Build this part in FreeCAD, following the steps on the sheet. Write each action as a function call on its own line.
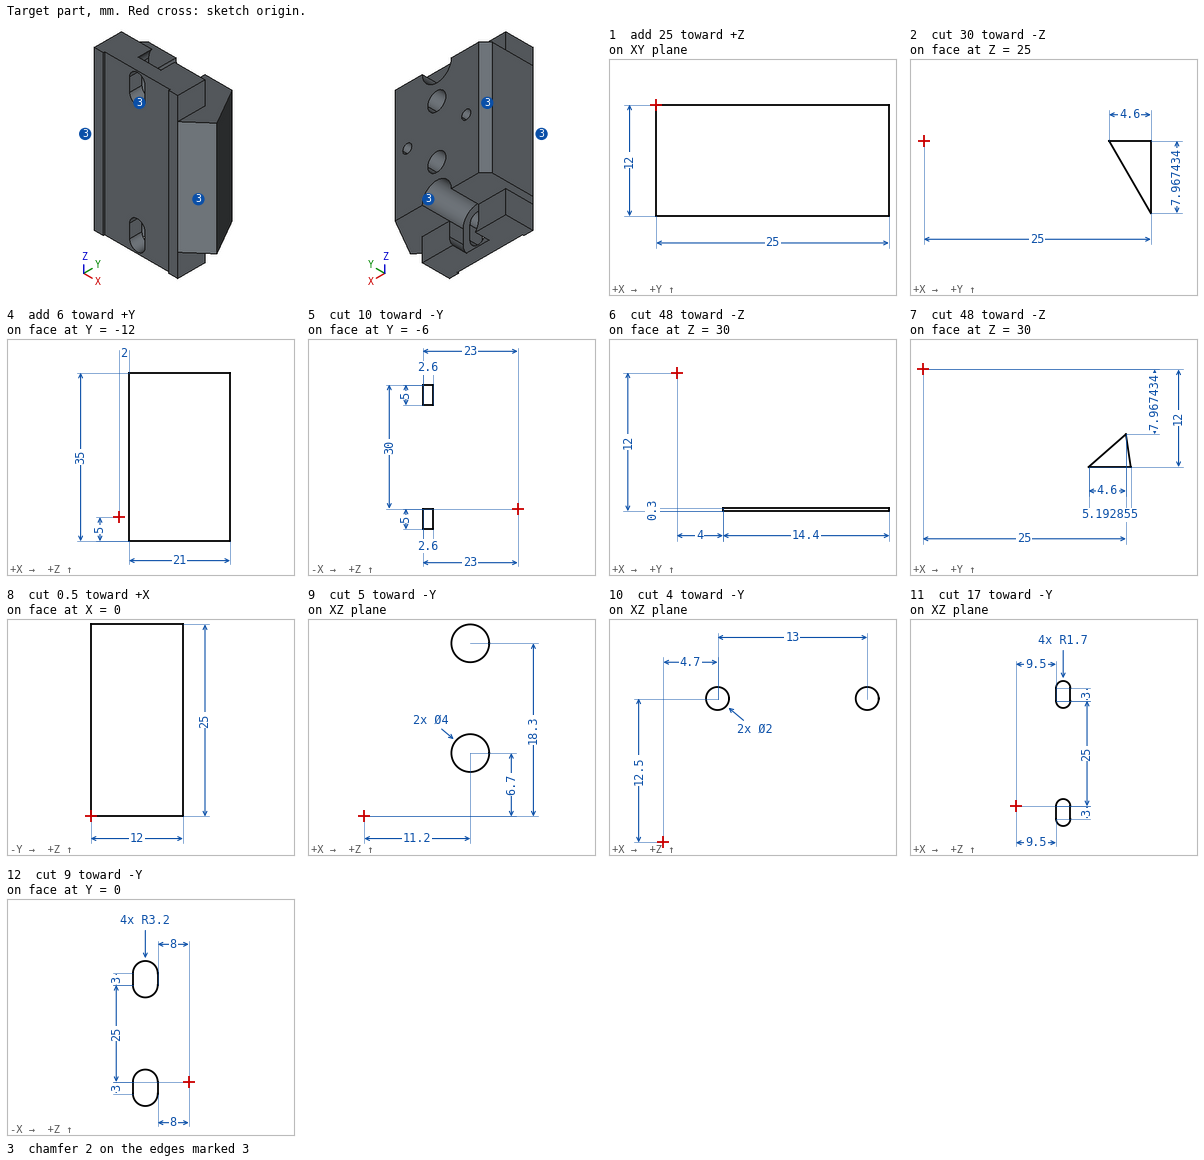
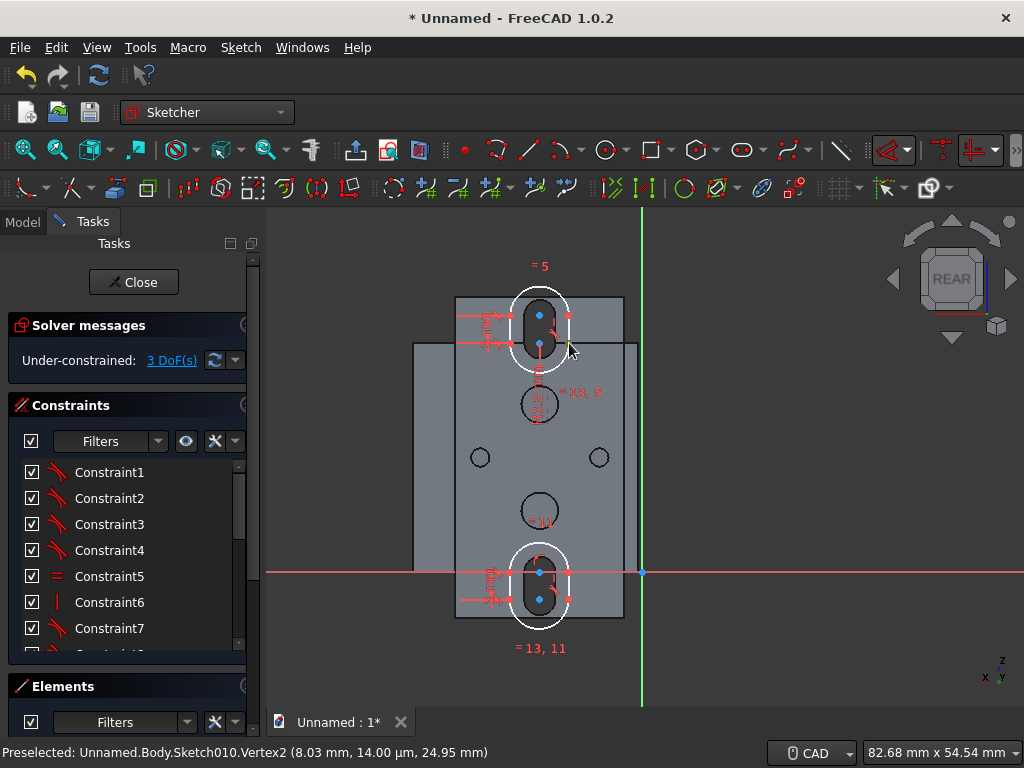
key(l)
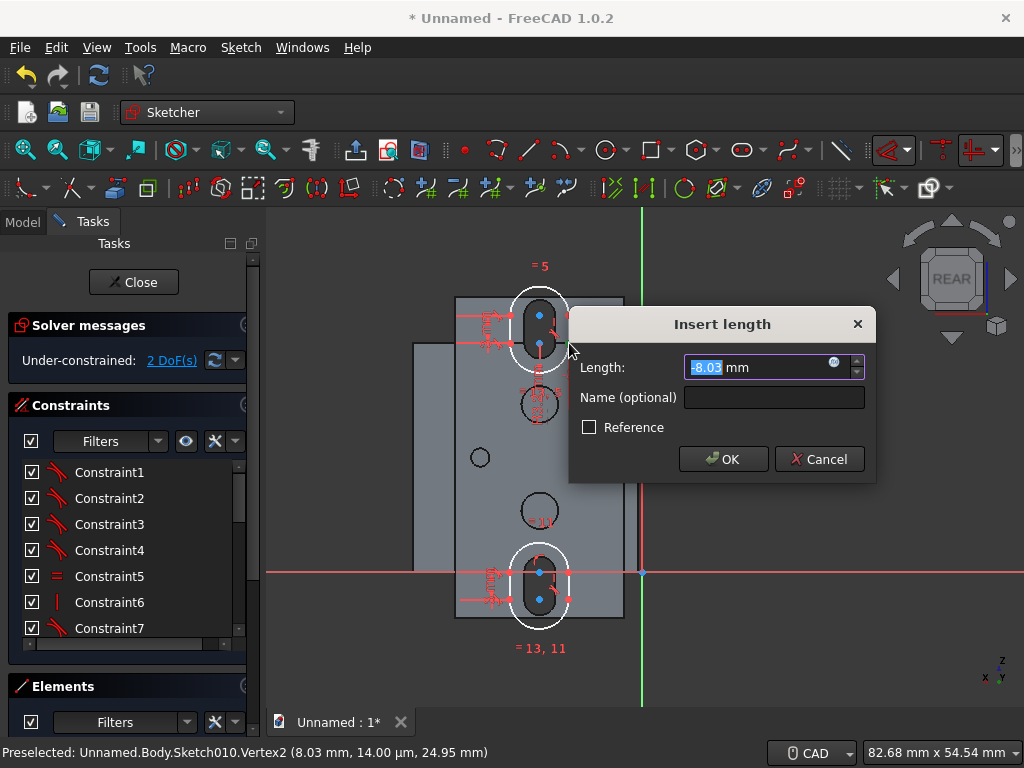
text(-8)
key(Return)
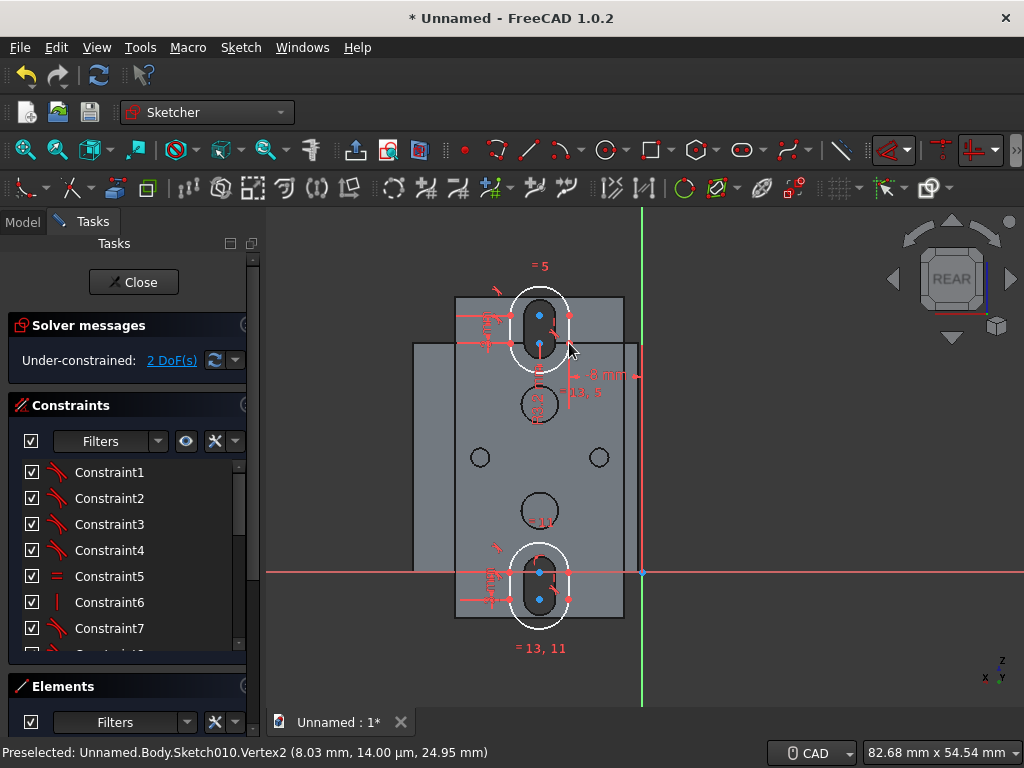
click(569, 600)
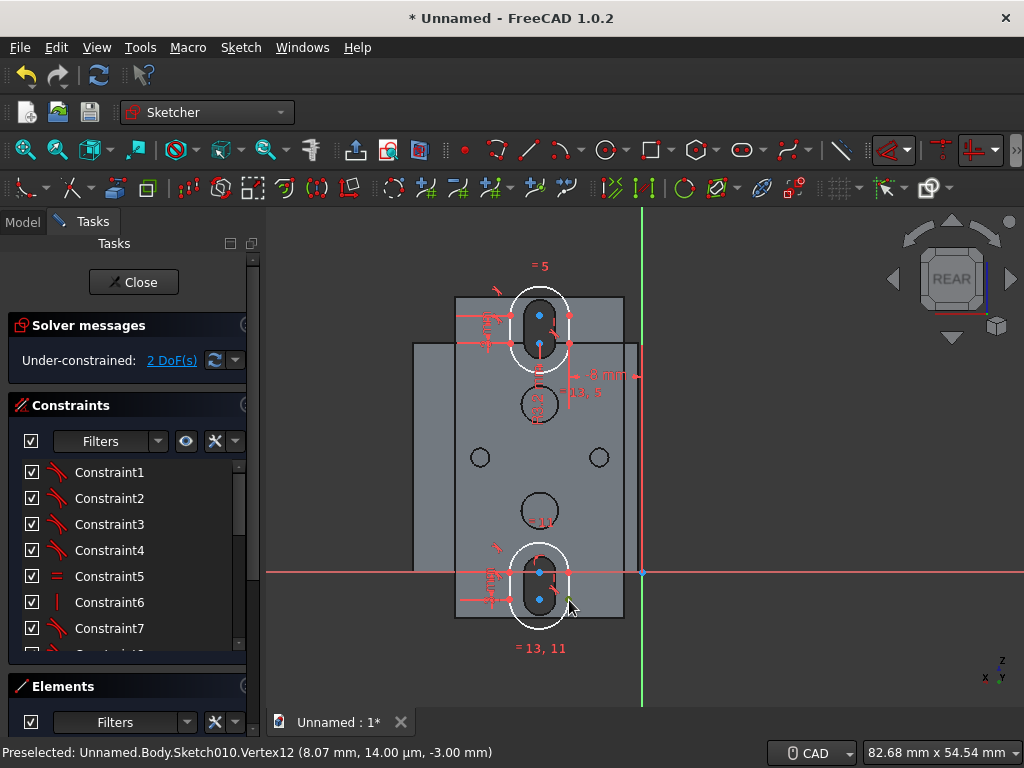
click(910, 150)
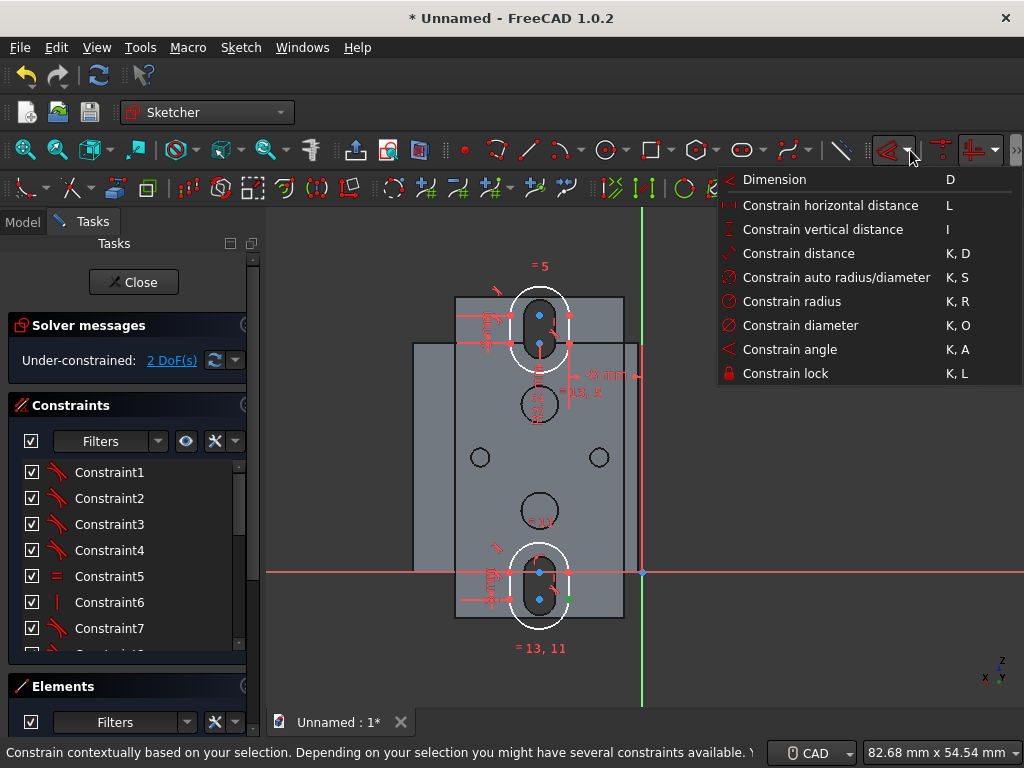
click(870, 205)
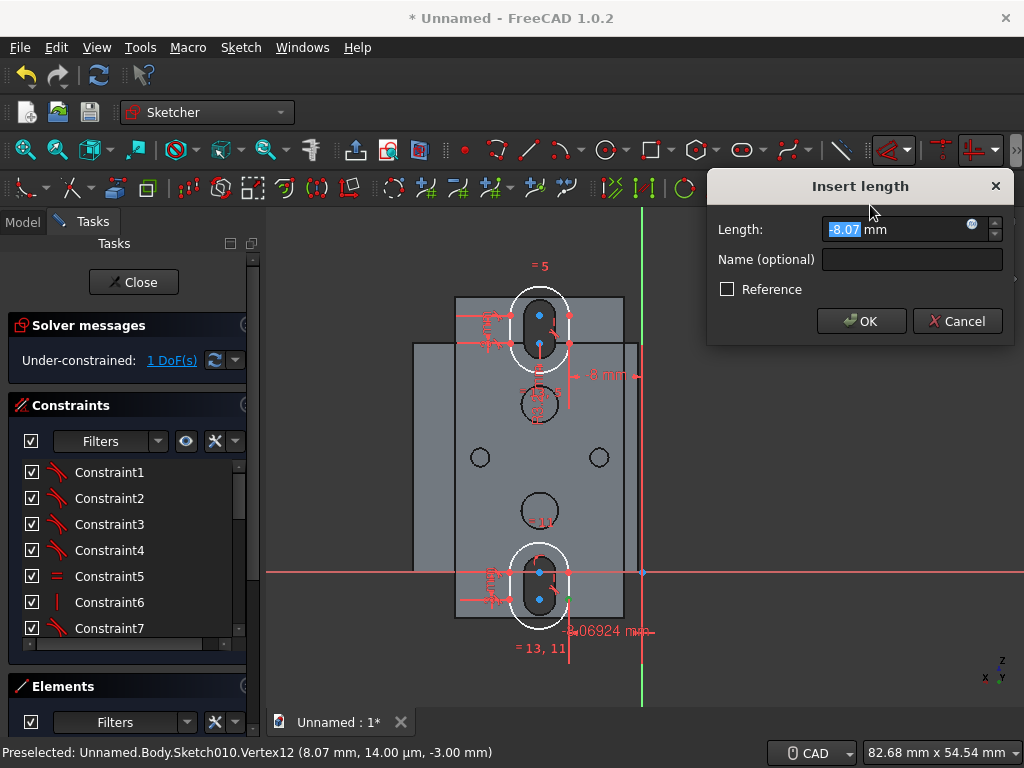
text(-8)
key(Return)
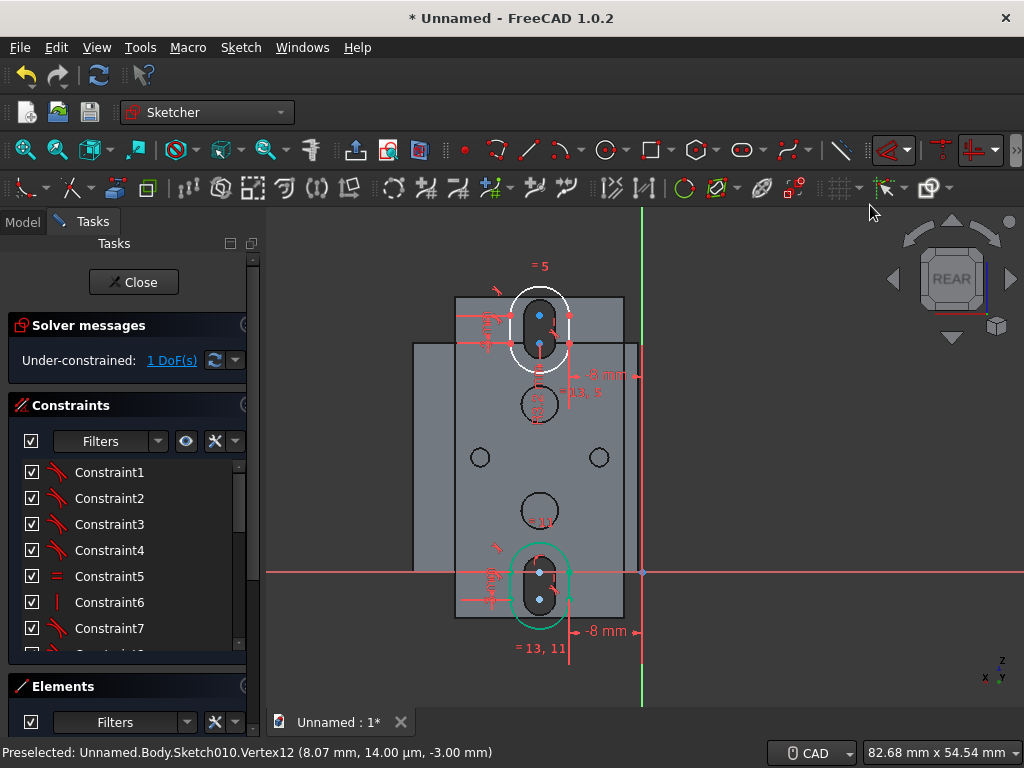
click(510, 343)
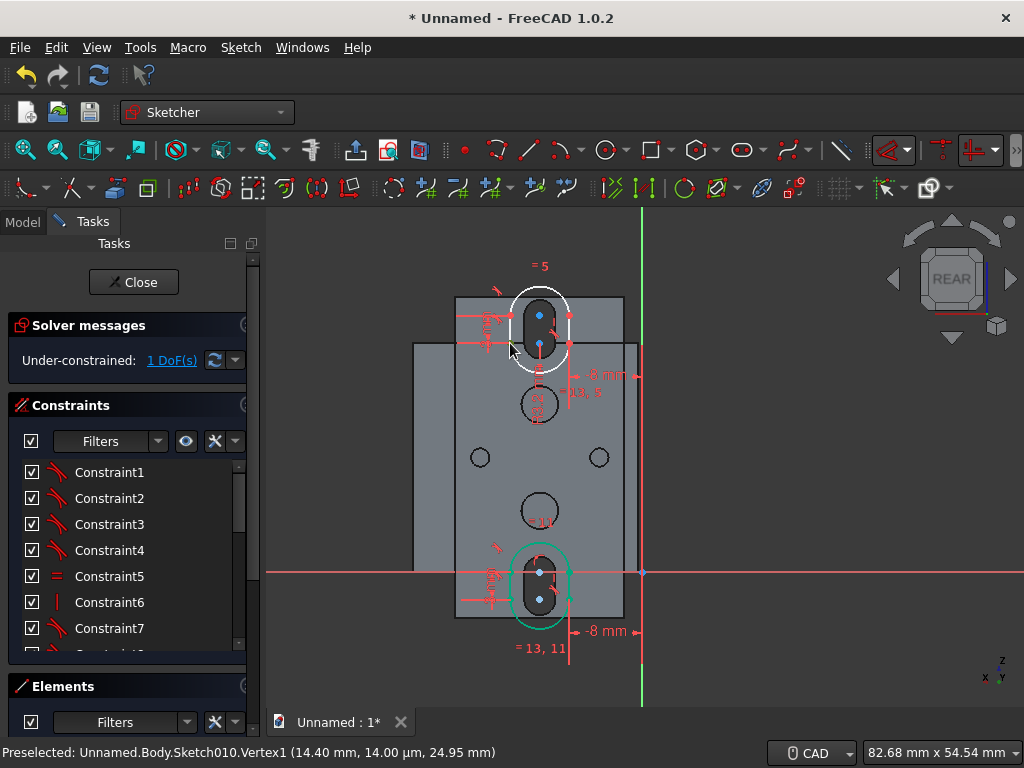
click(910, 150)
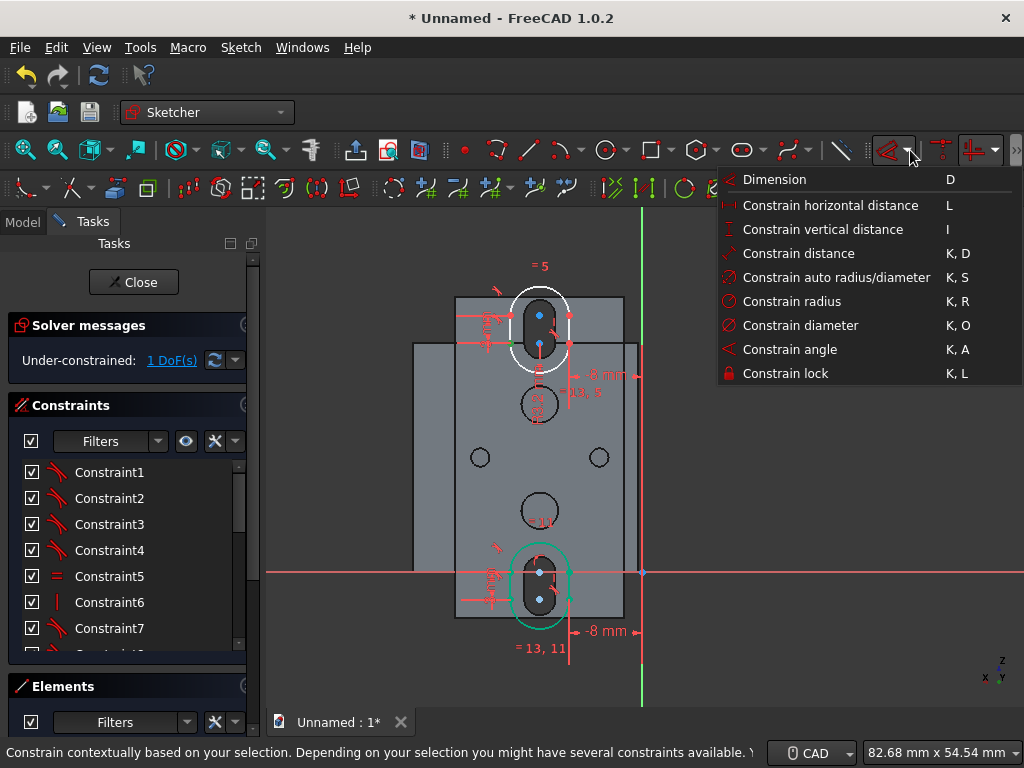
click(870, 229)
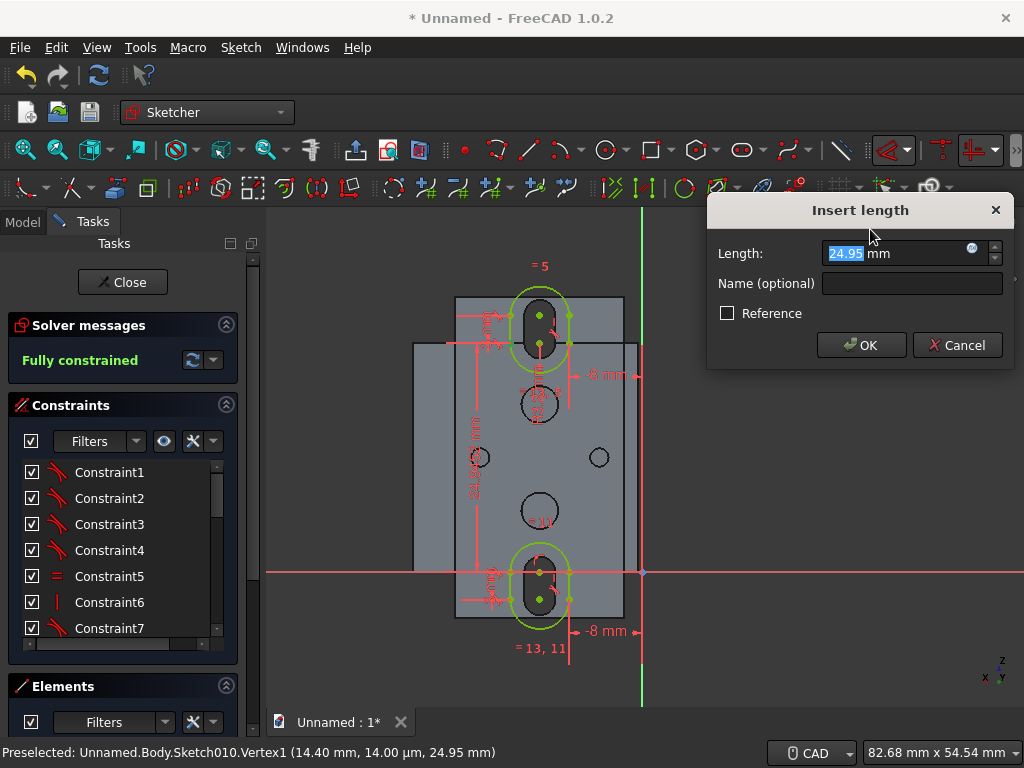
text(25)
key(Return)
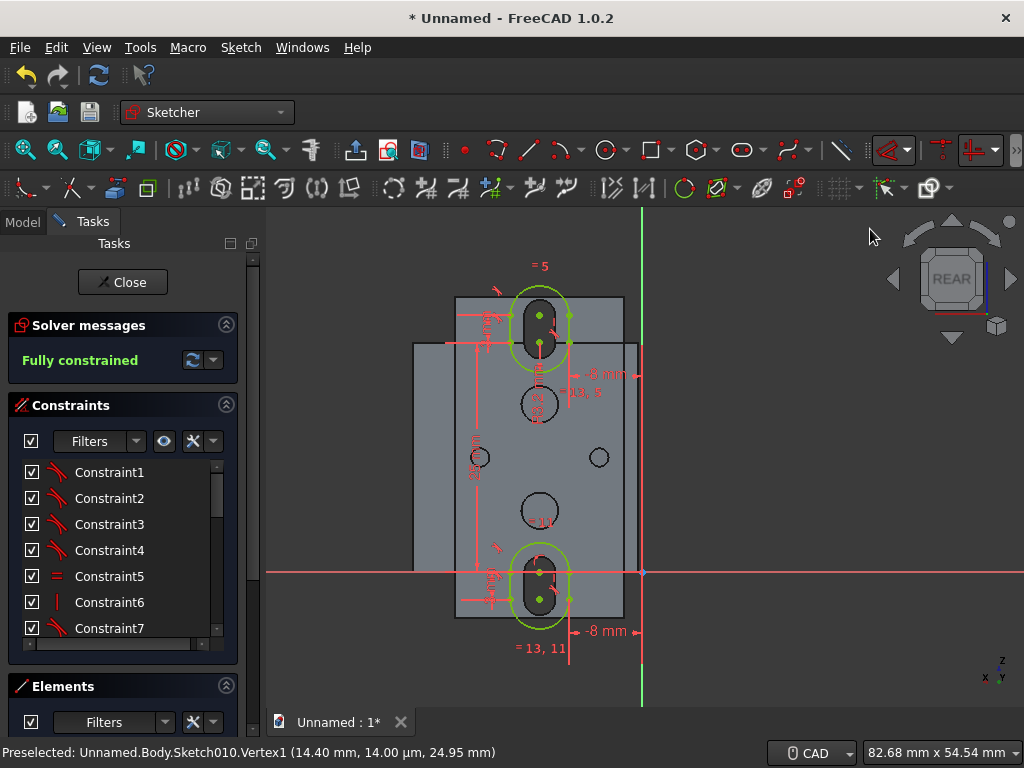
click(123, 282)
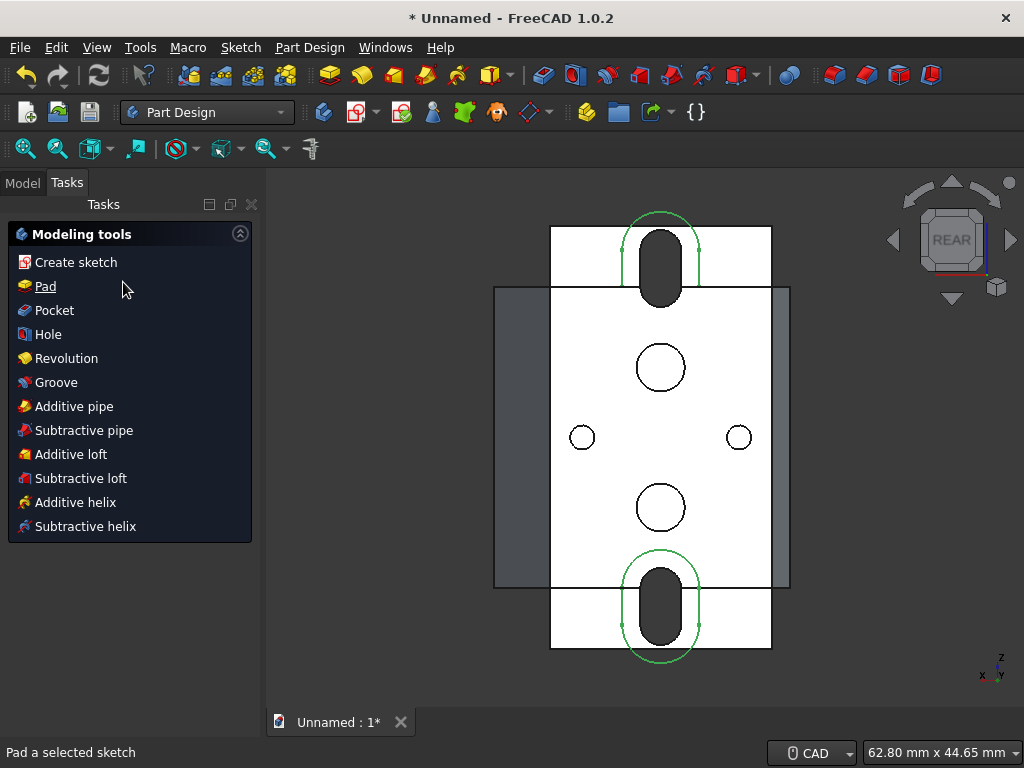
click(544, 76)